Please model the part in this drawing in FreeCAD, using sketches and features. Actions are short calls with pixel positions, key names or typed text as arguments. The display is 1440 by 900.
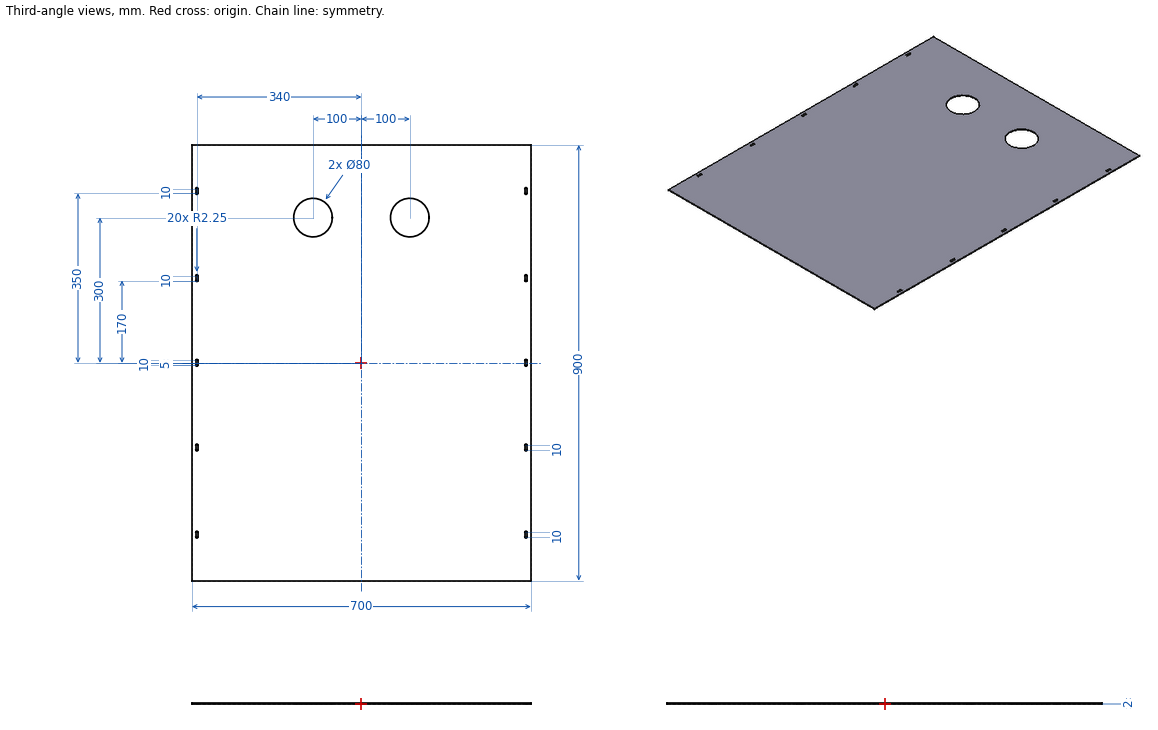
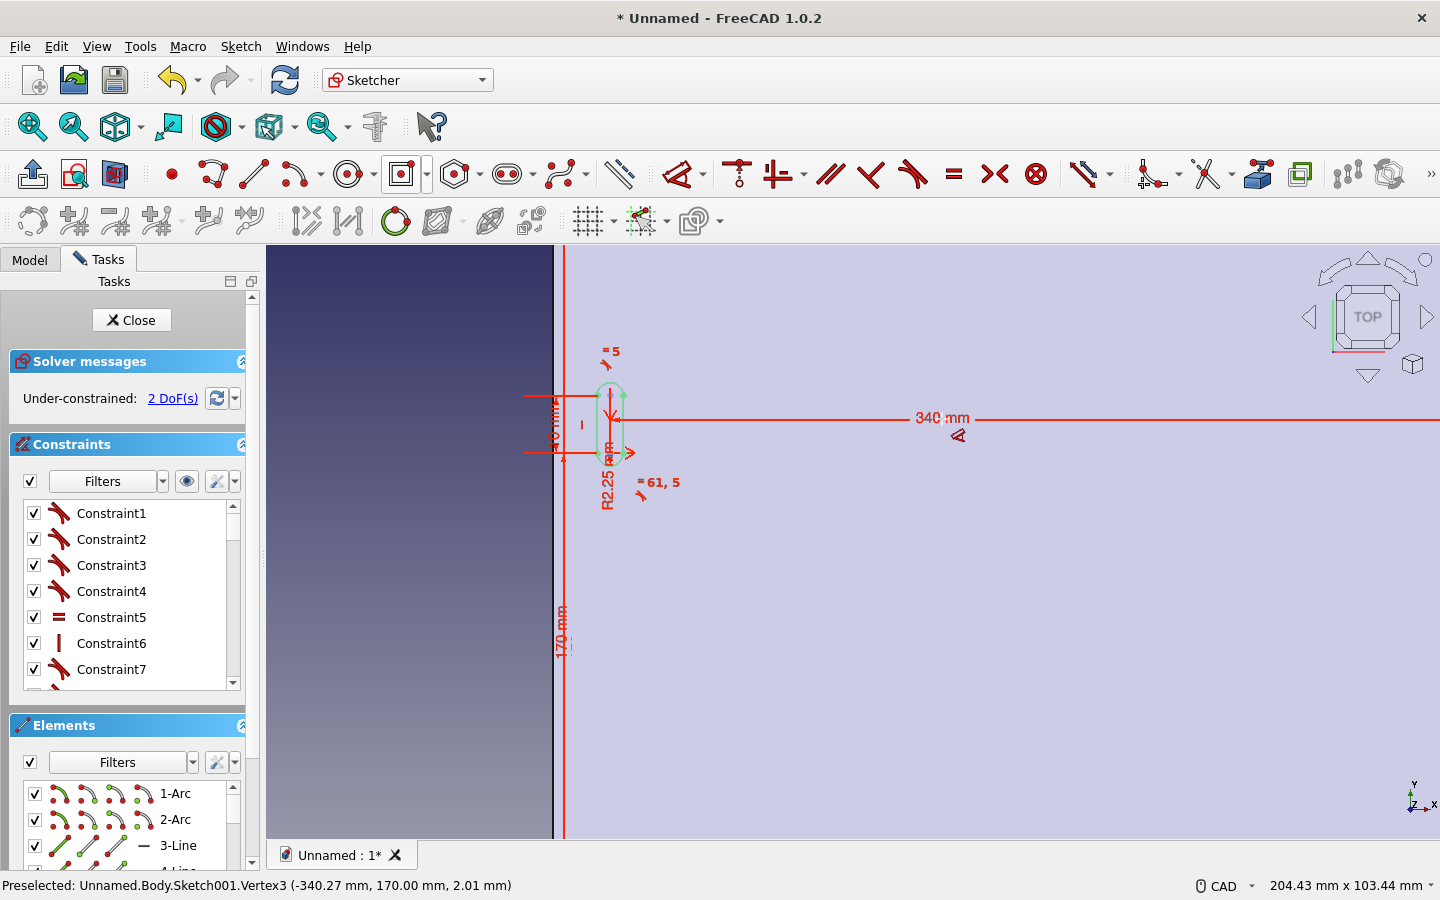
scroll(607, 453, down, 12)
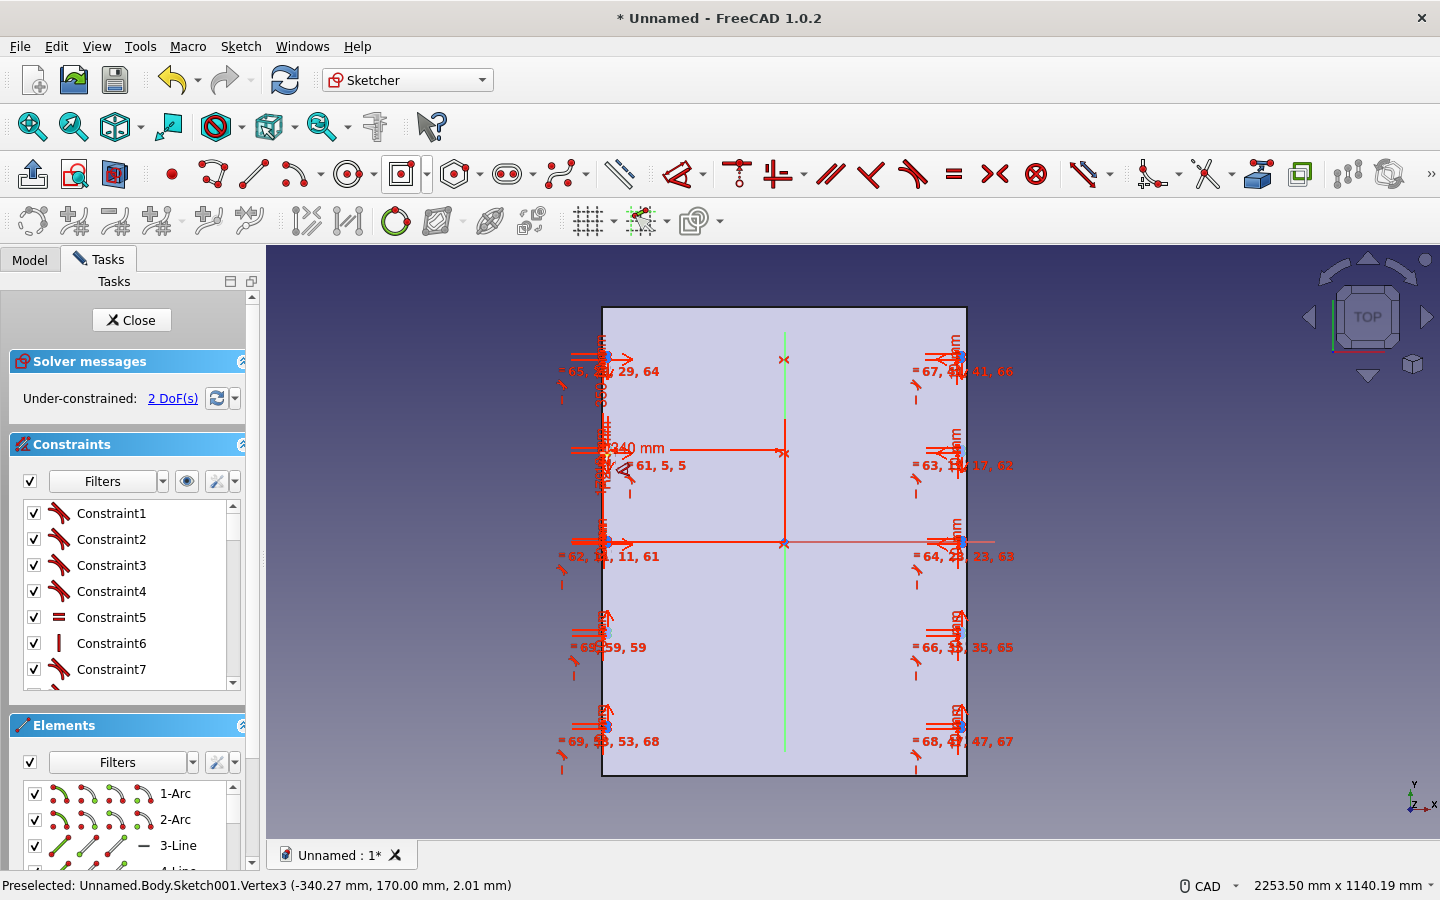
scroll(607, 544, up, 12)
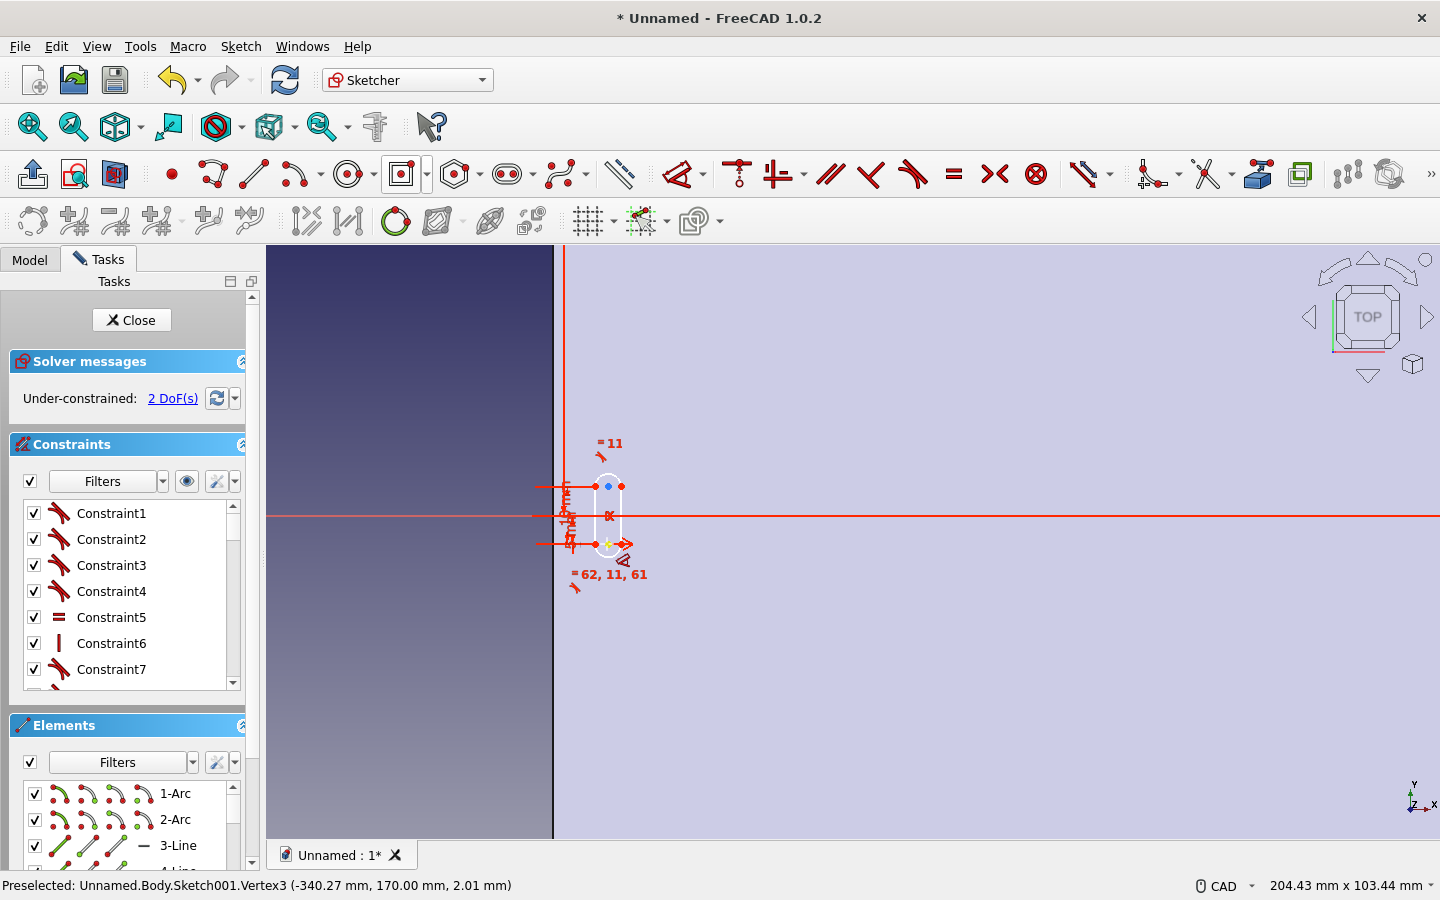
click(608, 544)
click(942, 578)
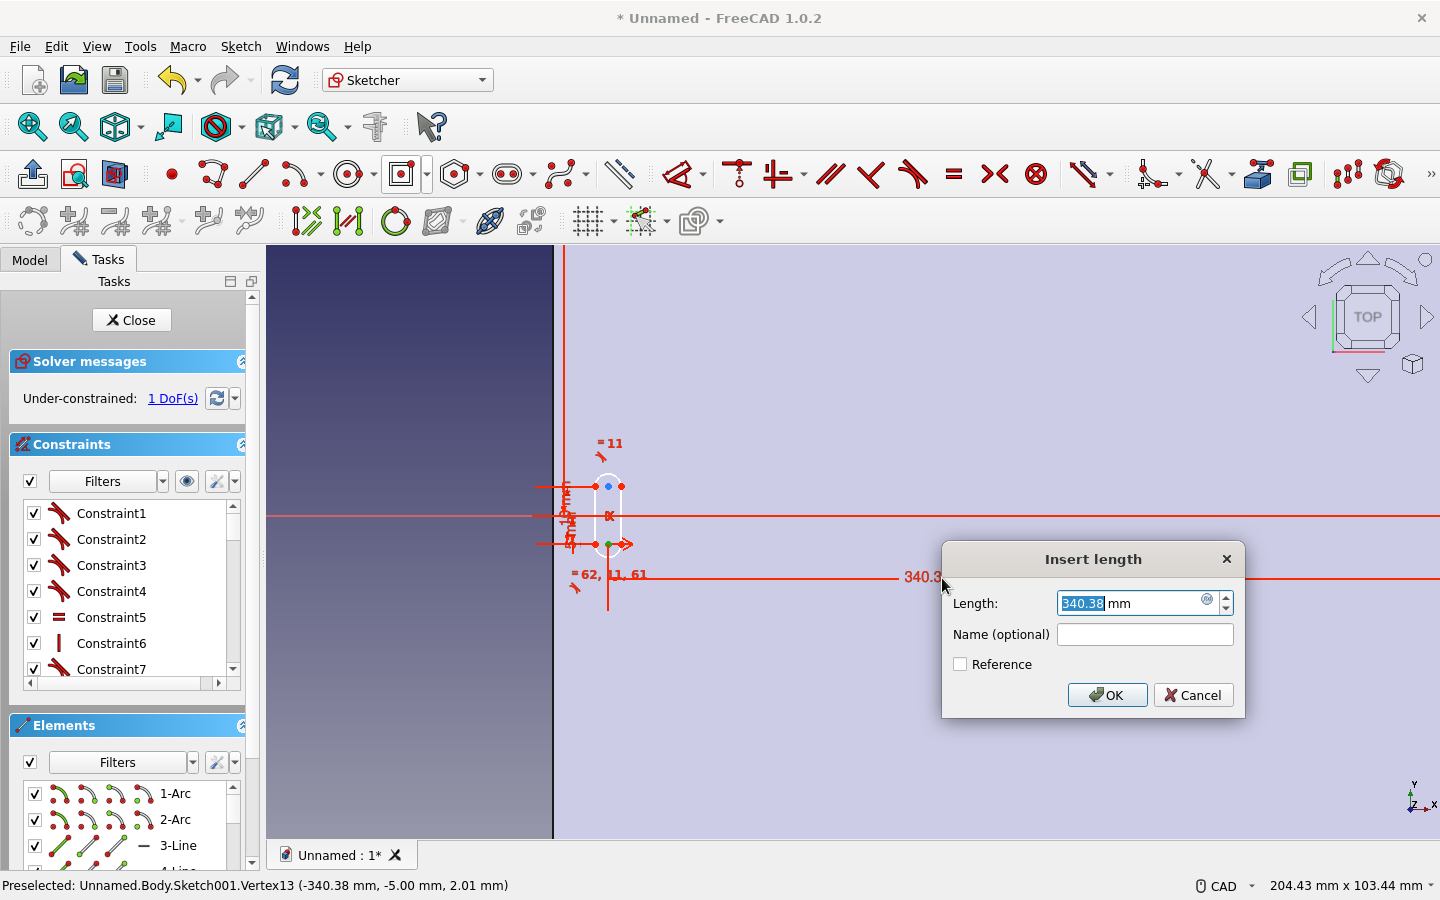
text(340)
key(Return)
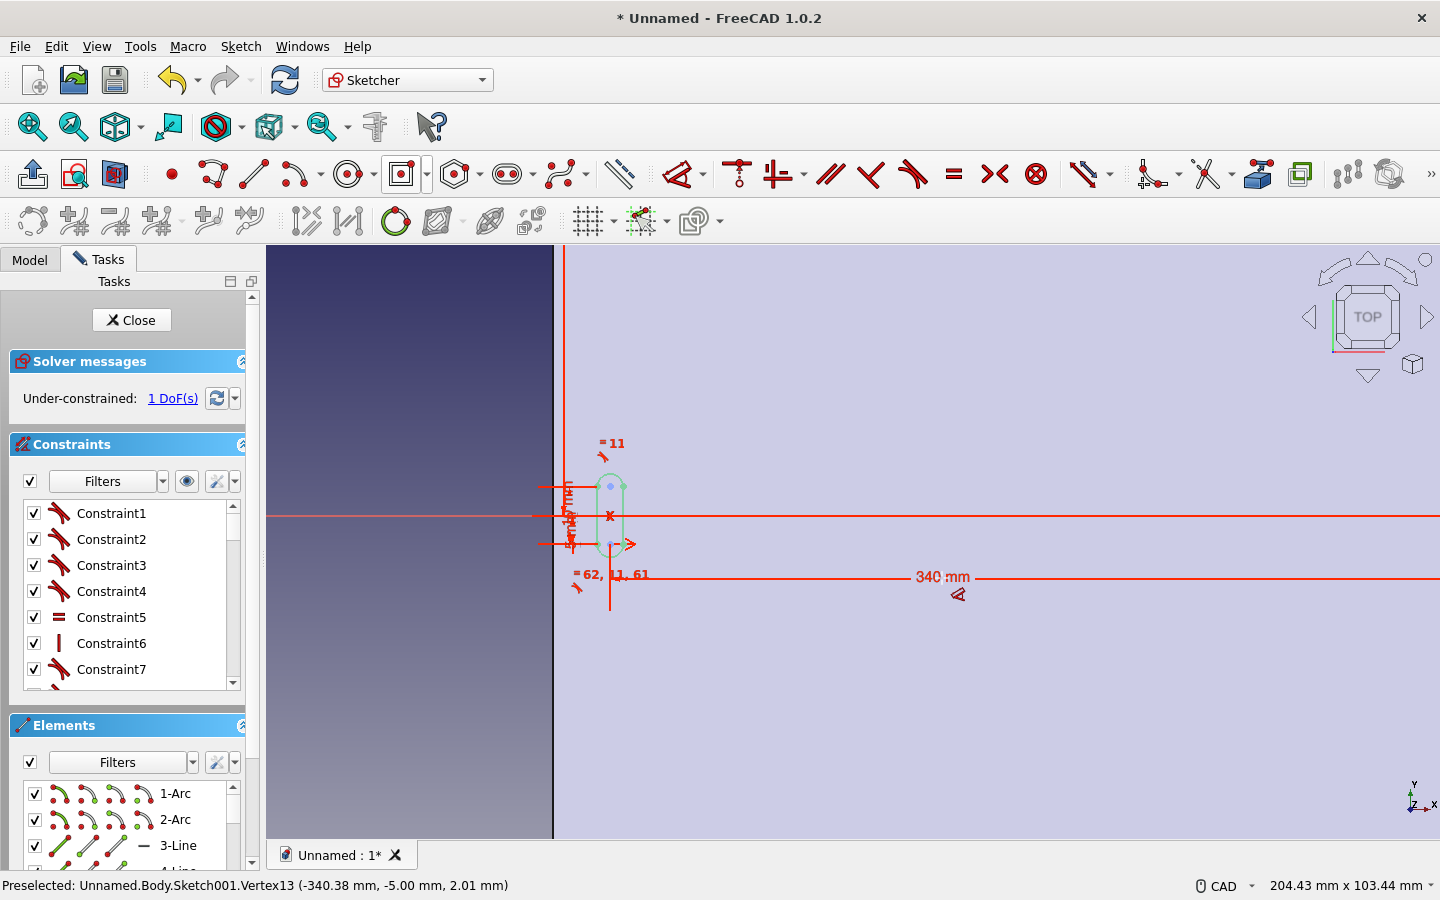
scroll(607, 545, down, 12)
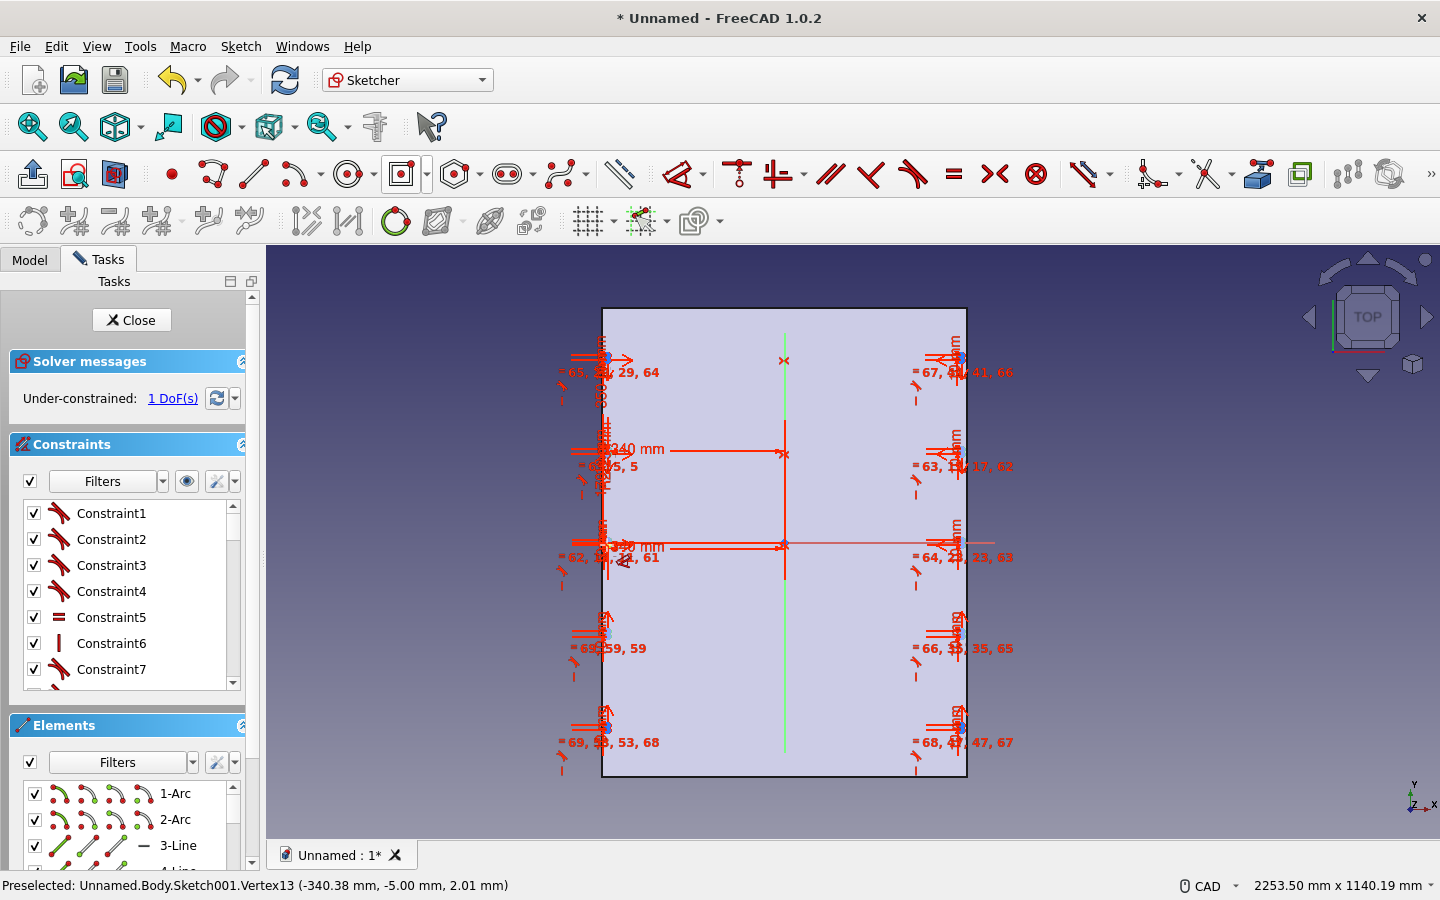
scroll(608, 360, up, 12)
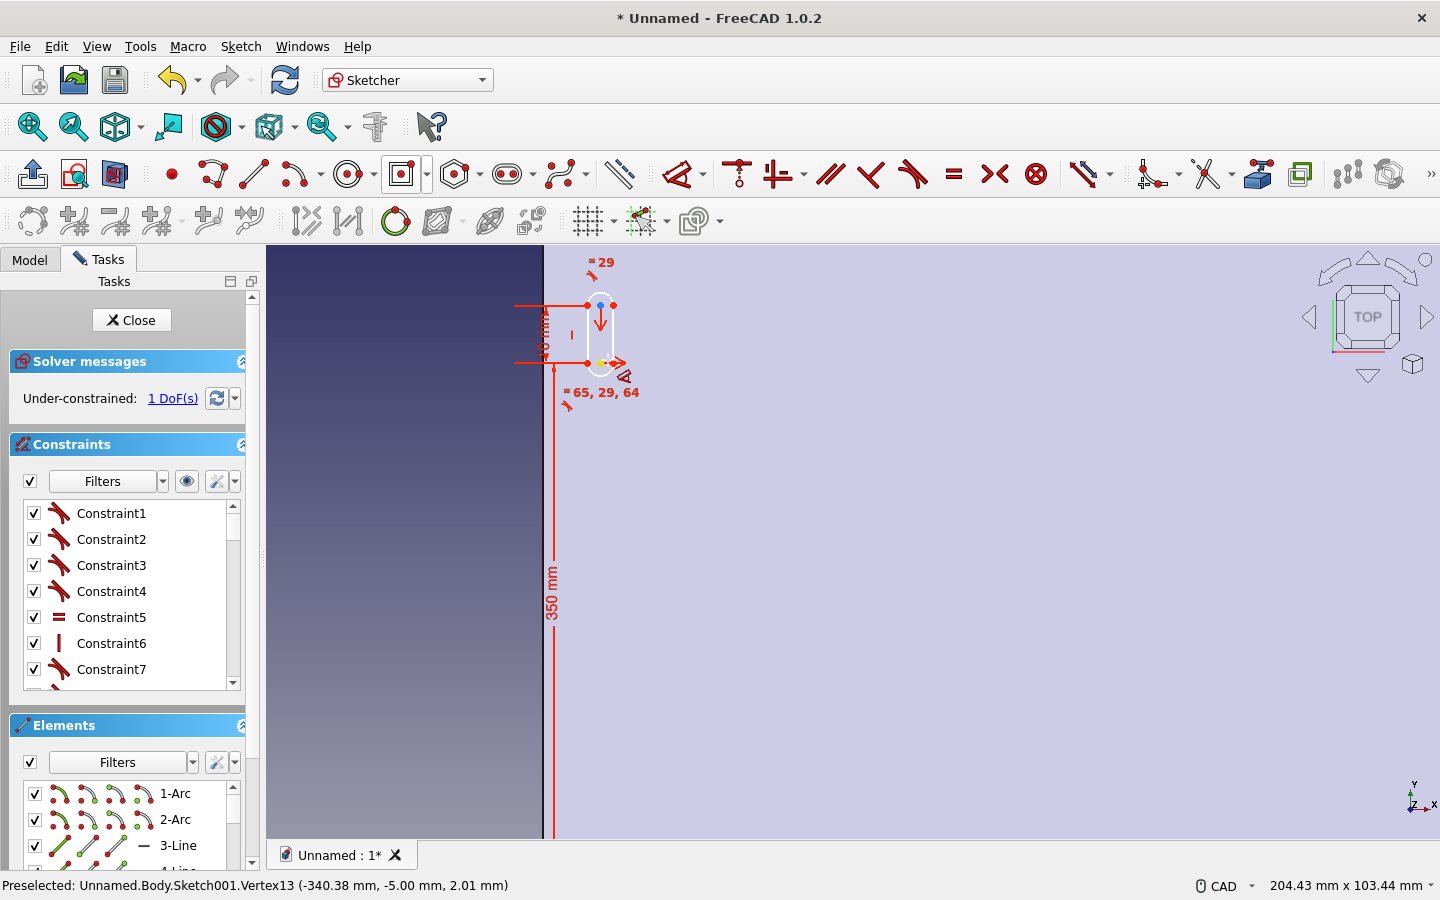
click(601, 363)
click(938, 329)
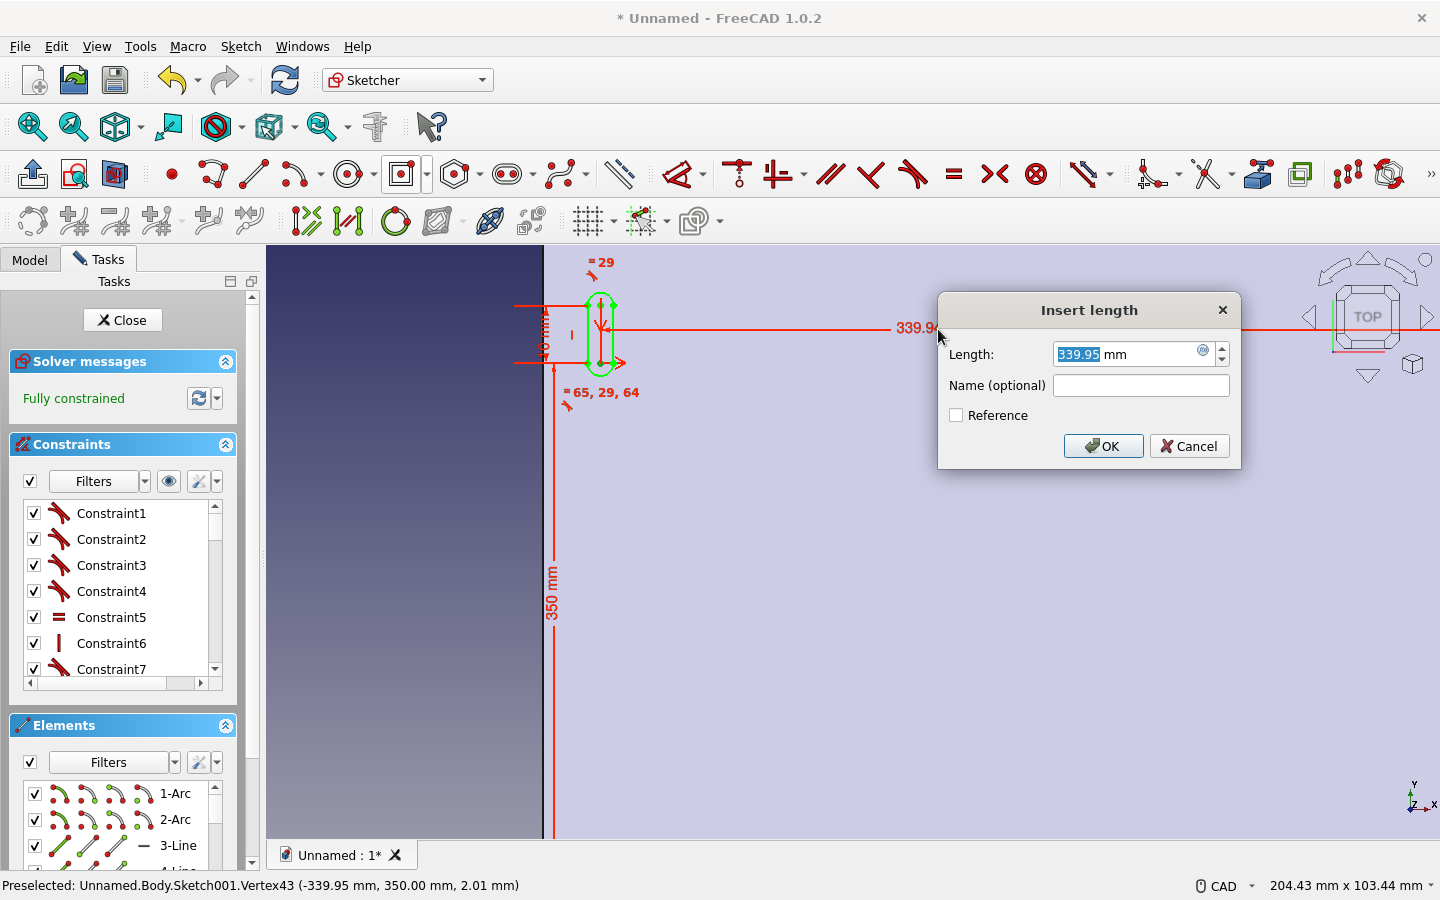
text(340)
key(Return)
key(Escape)